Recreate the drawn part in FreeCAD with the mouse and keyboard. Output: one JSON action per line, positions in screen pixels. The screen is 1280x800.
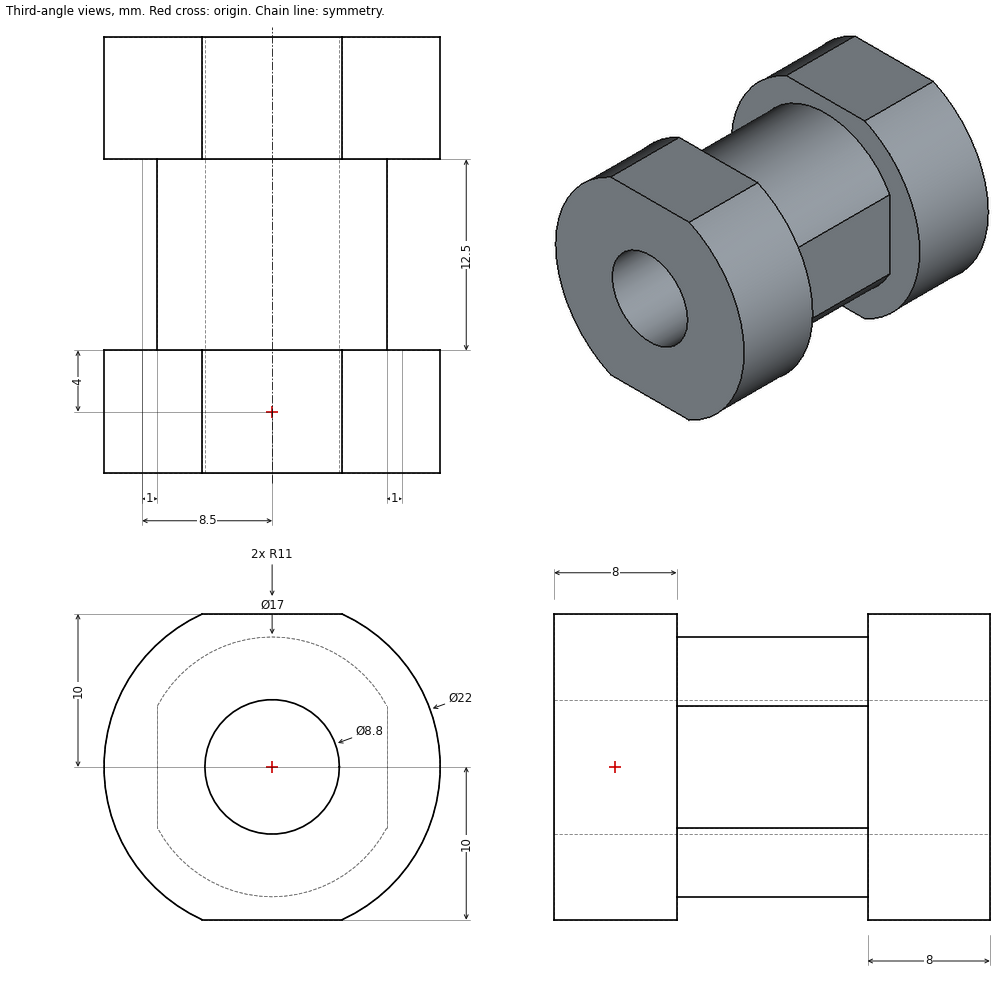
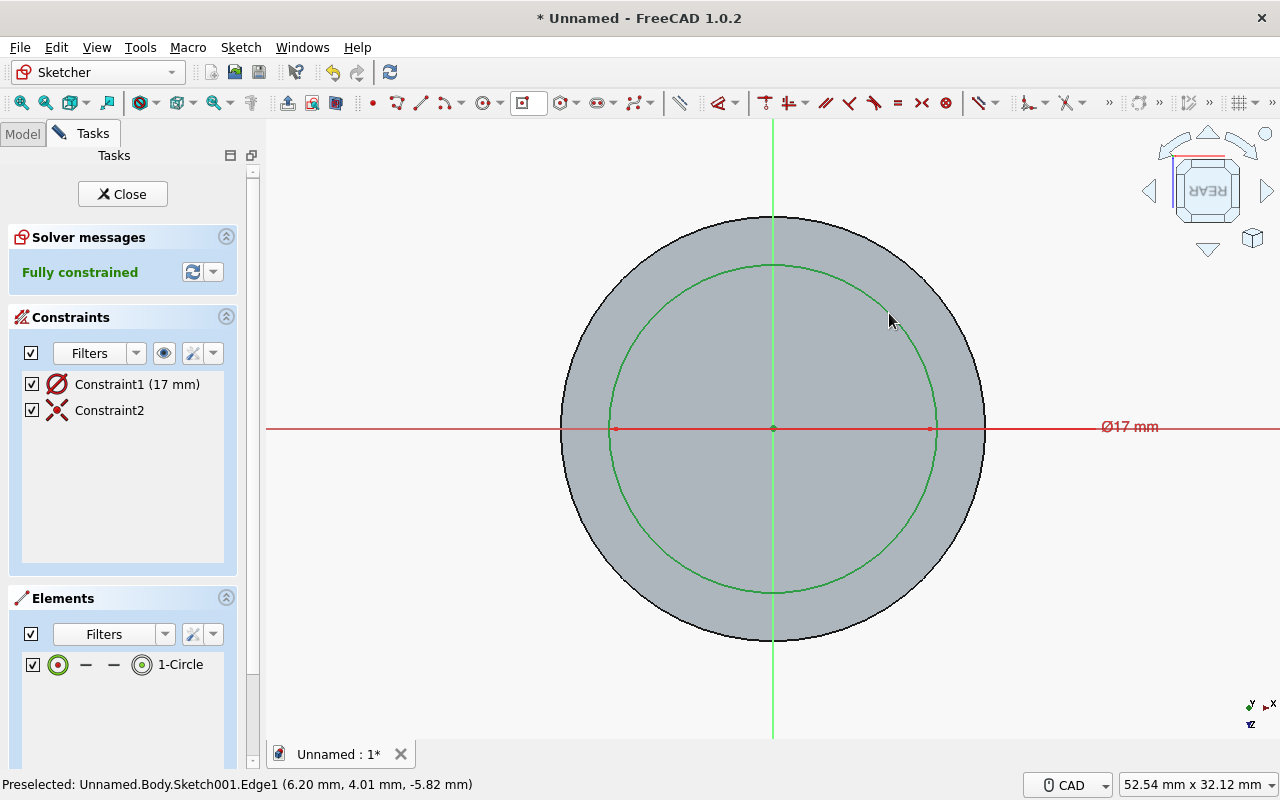
{"action": "left_click", "coordinate": [123, 194]}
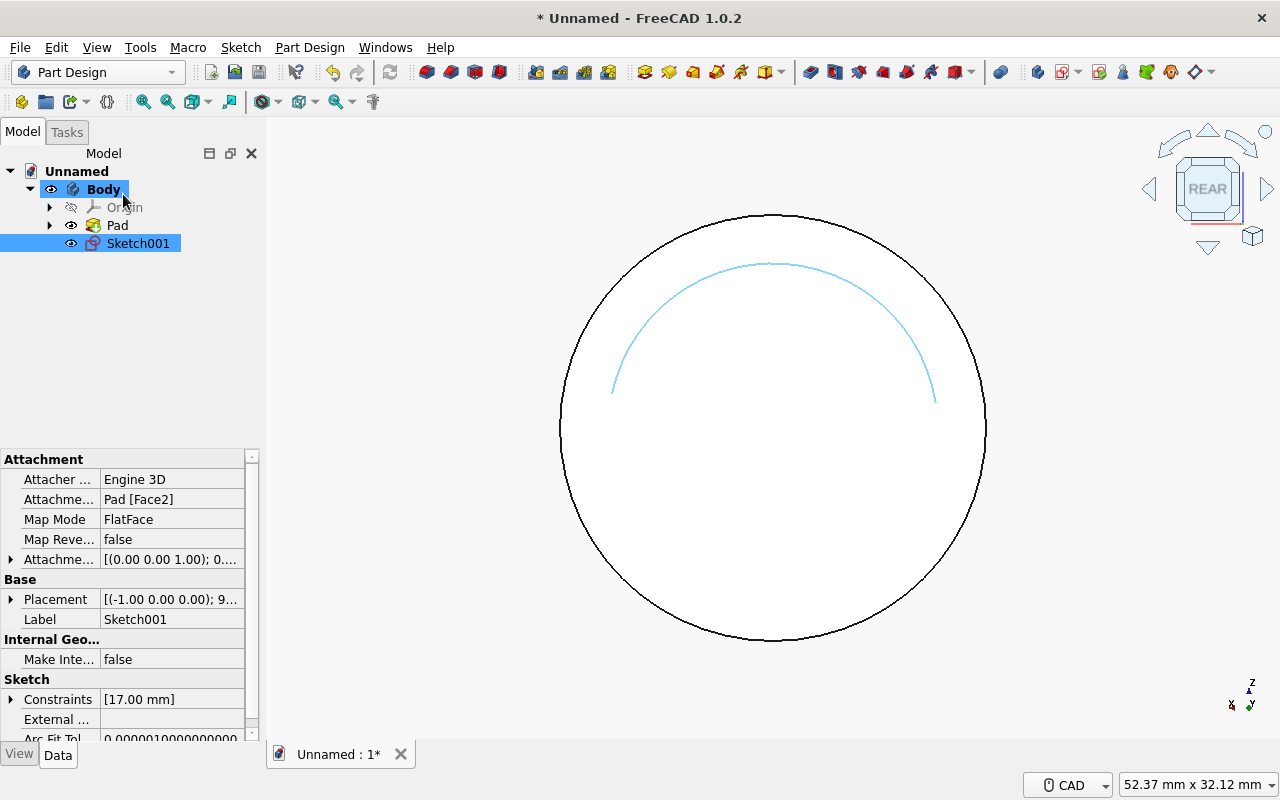
{"action": "left_click", "coordinate": [646, 72]}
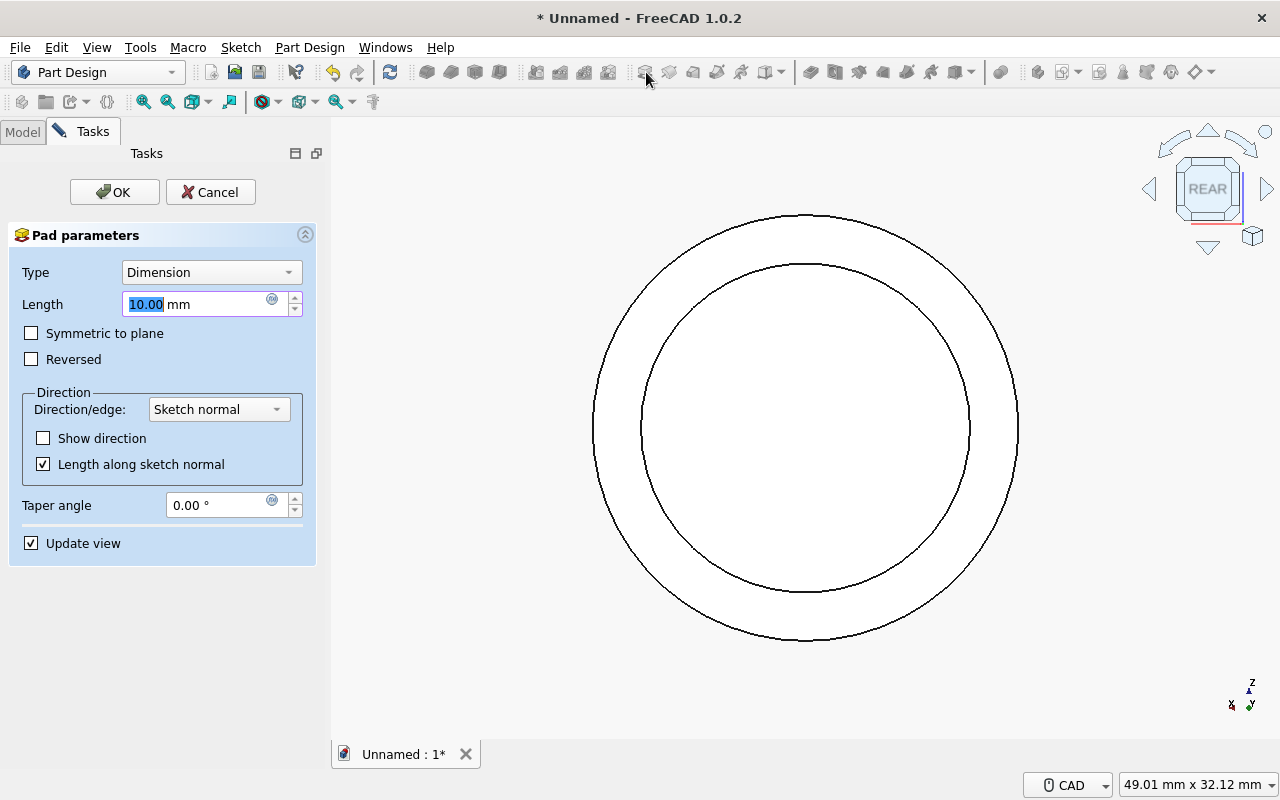
{"action": "type", "text": "12.5"}
{"action": "key", "text": "Tab"}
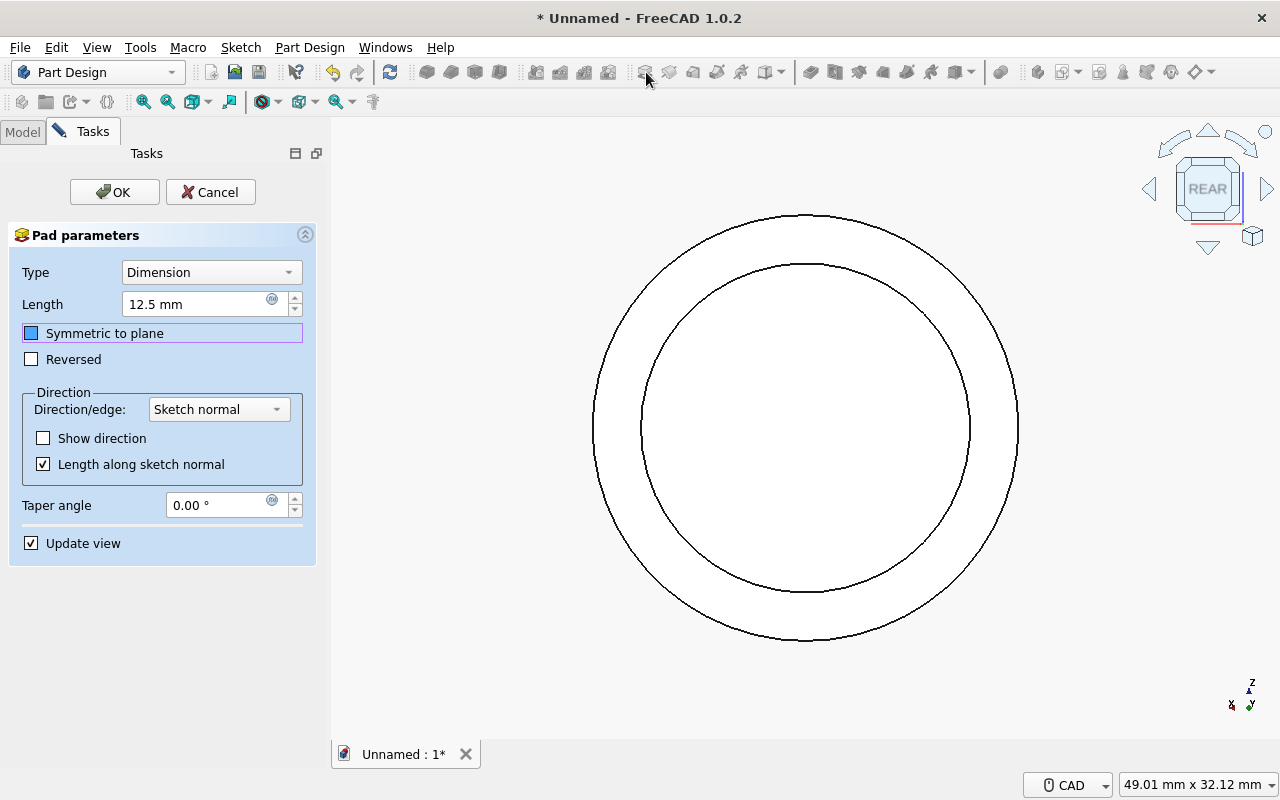
{"action": "left_click", "coordinate": [115, 192]}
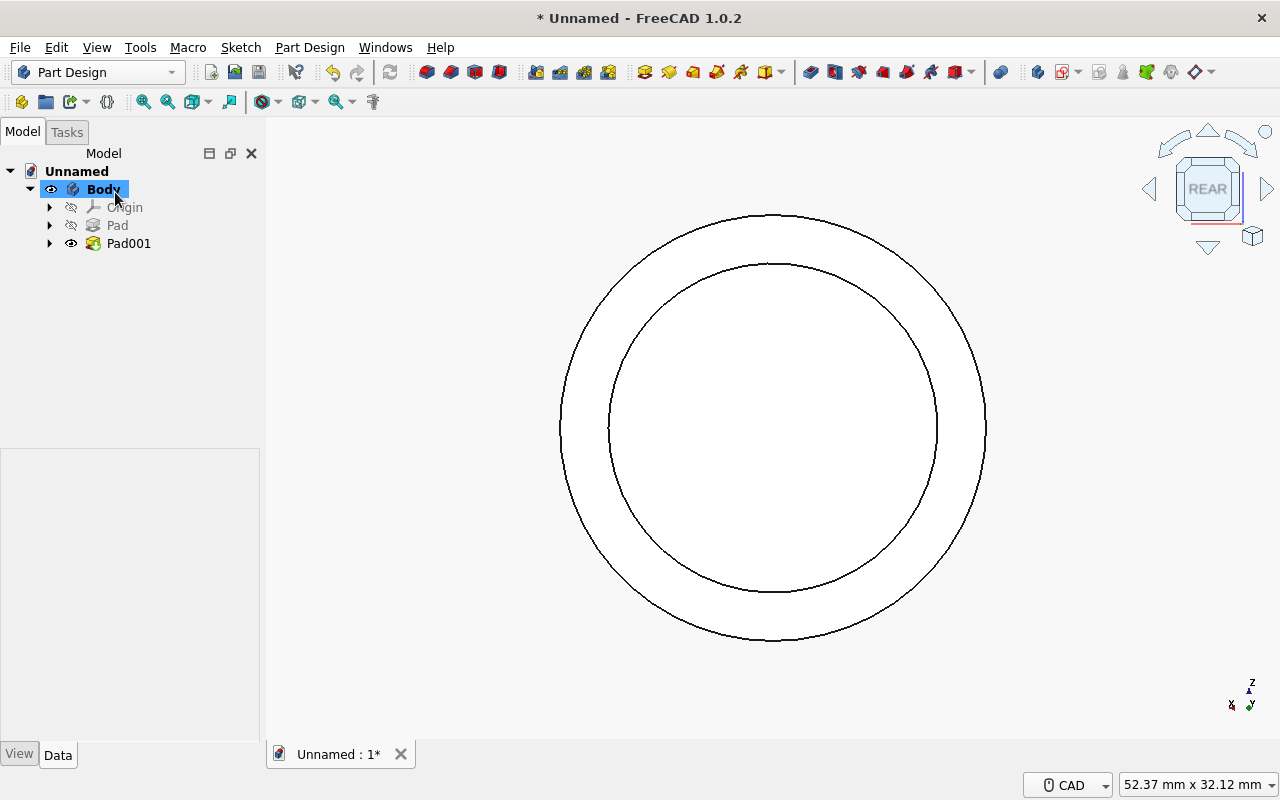
{"action": "left_click", "coordinate": [50, 207]}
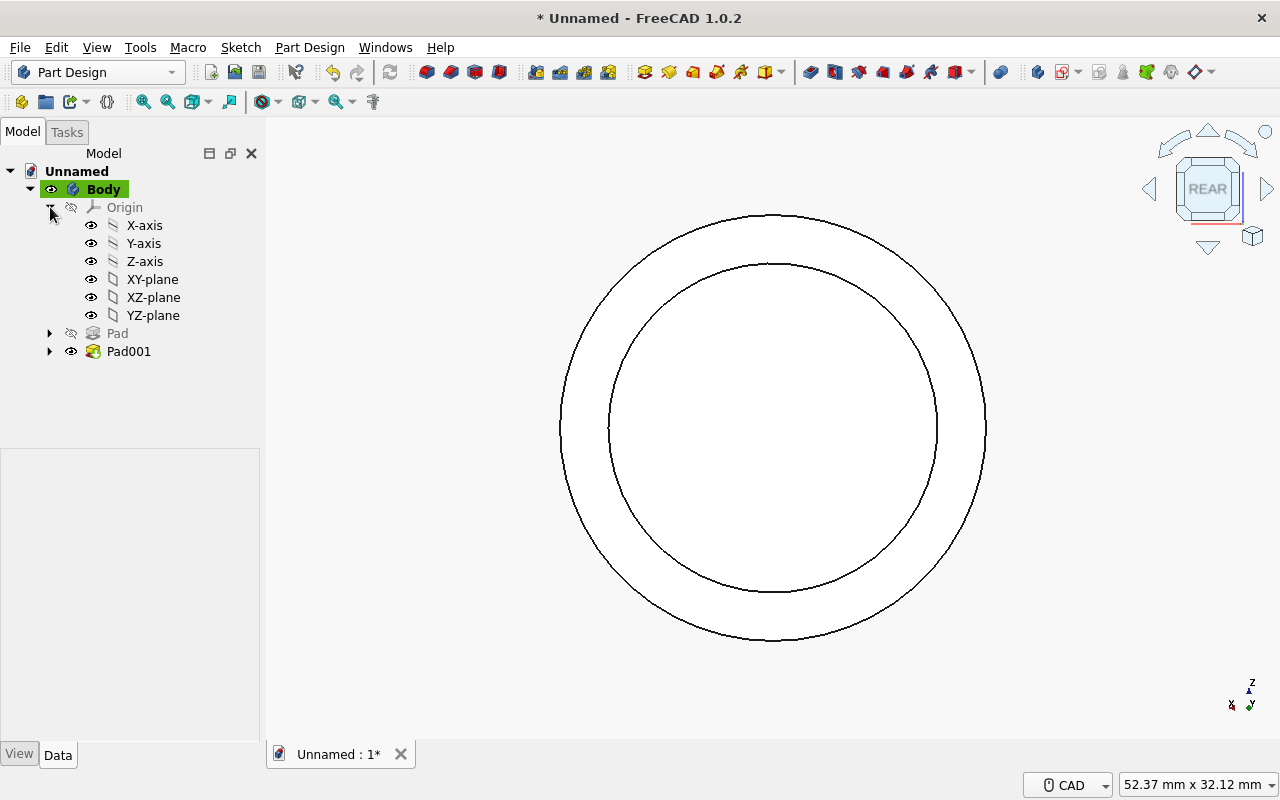
{"action": "left_click", "coordinate": [136, 297]}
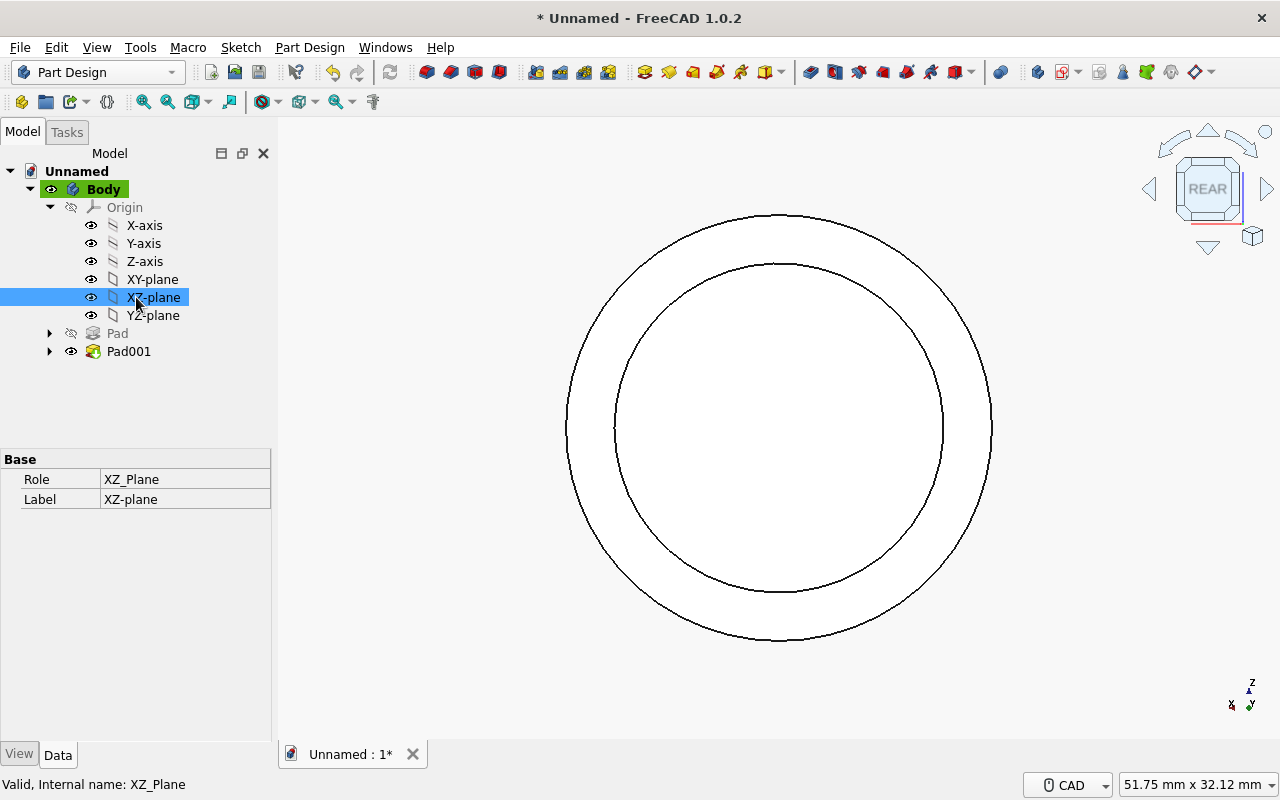
{"action": "left_click", "coordinate": [1196, 72]}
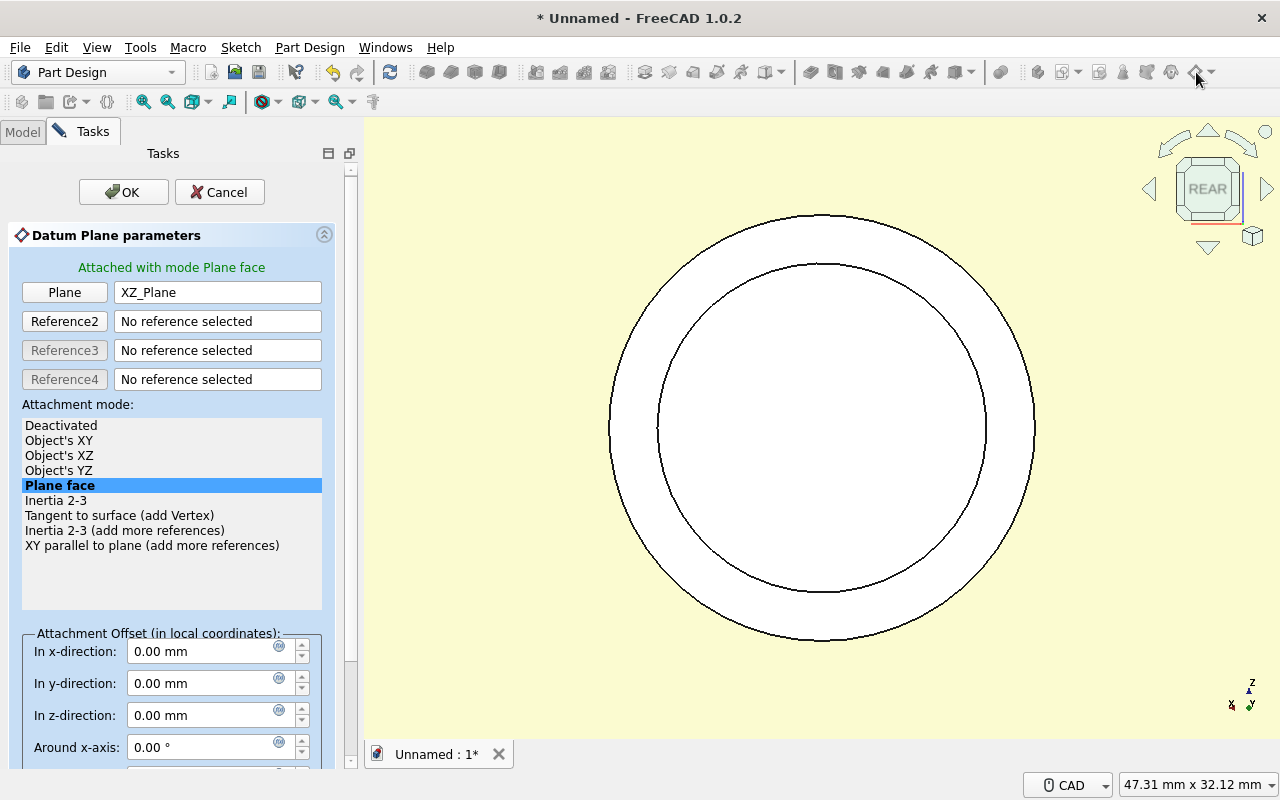
{"action": "triple_click", "coordinate": [210, 715]}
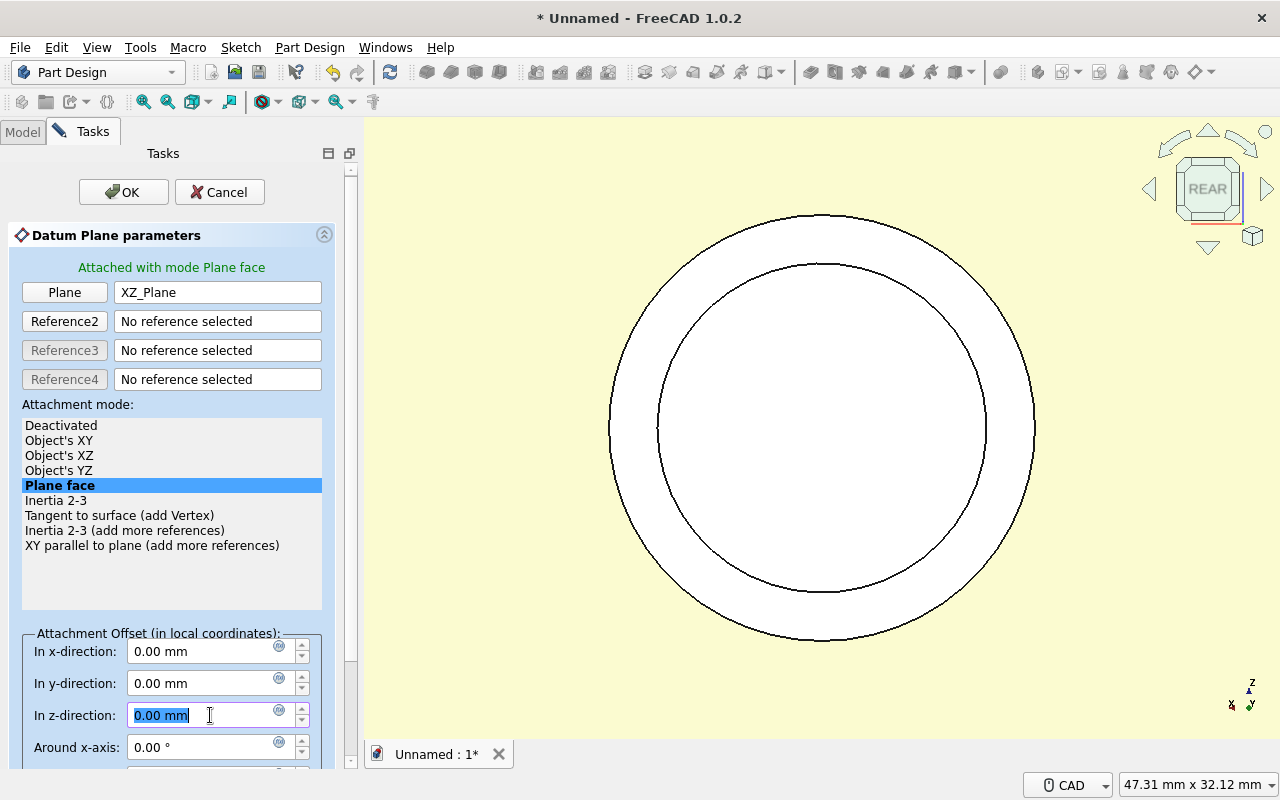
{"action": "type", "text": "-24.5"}
{"action": "key", "text": "Tab"}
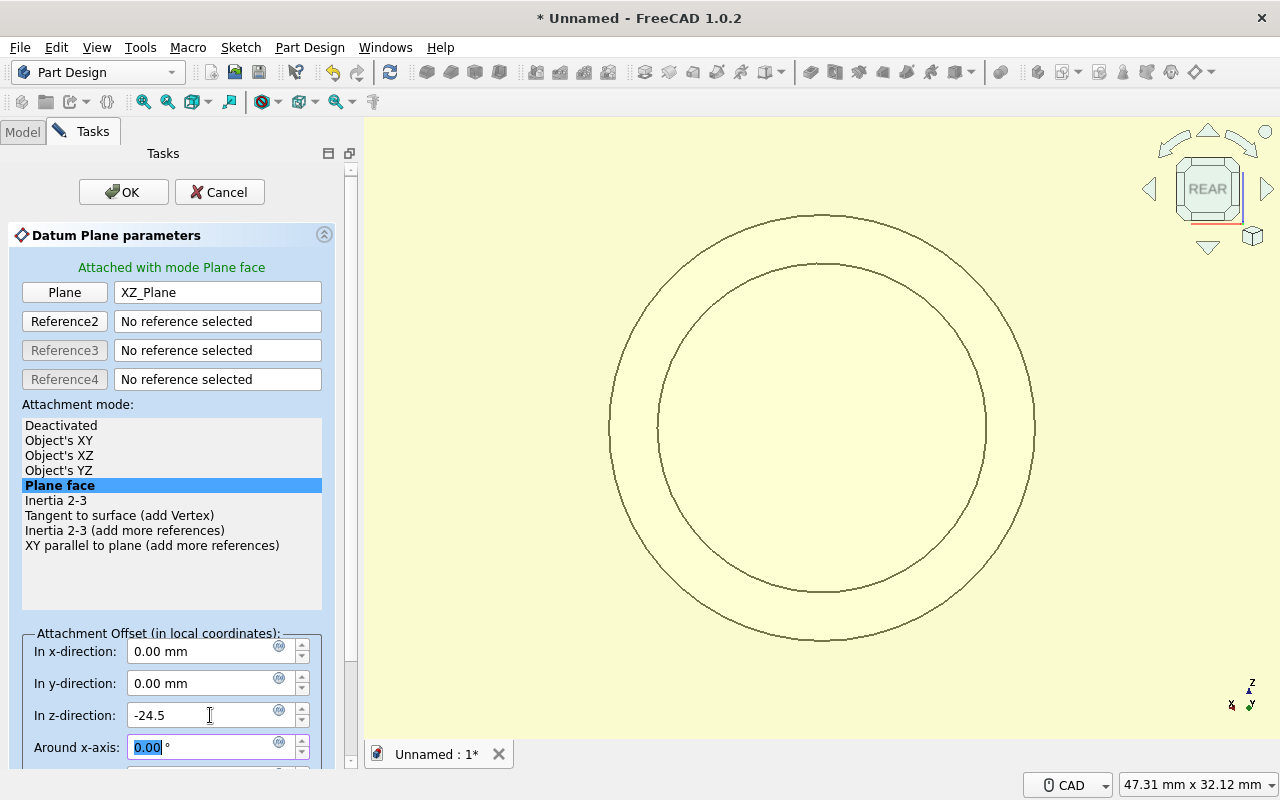
{"action": "left_click", "coordinate": [124, 192]}